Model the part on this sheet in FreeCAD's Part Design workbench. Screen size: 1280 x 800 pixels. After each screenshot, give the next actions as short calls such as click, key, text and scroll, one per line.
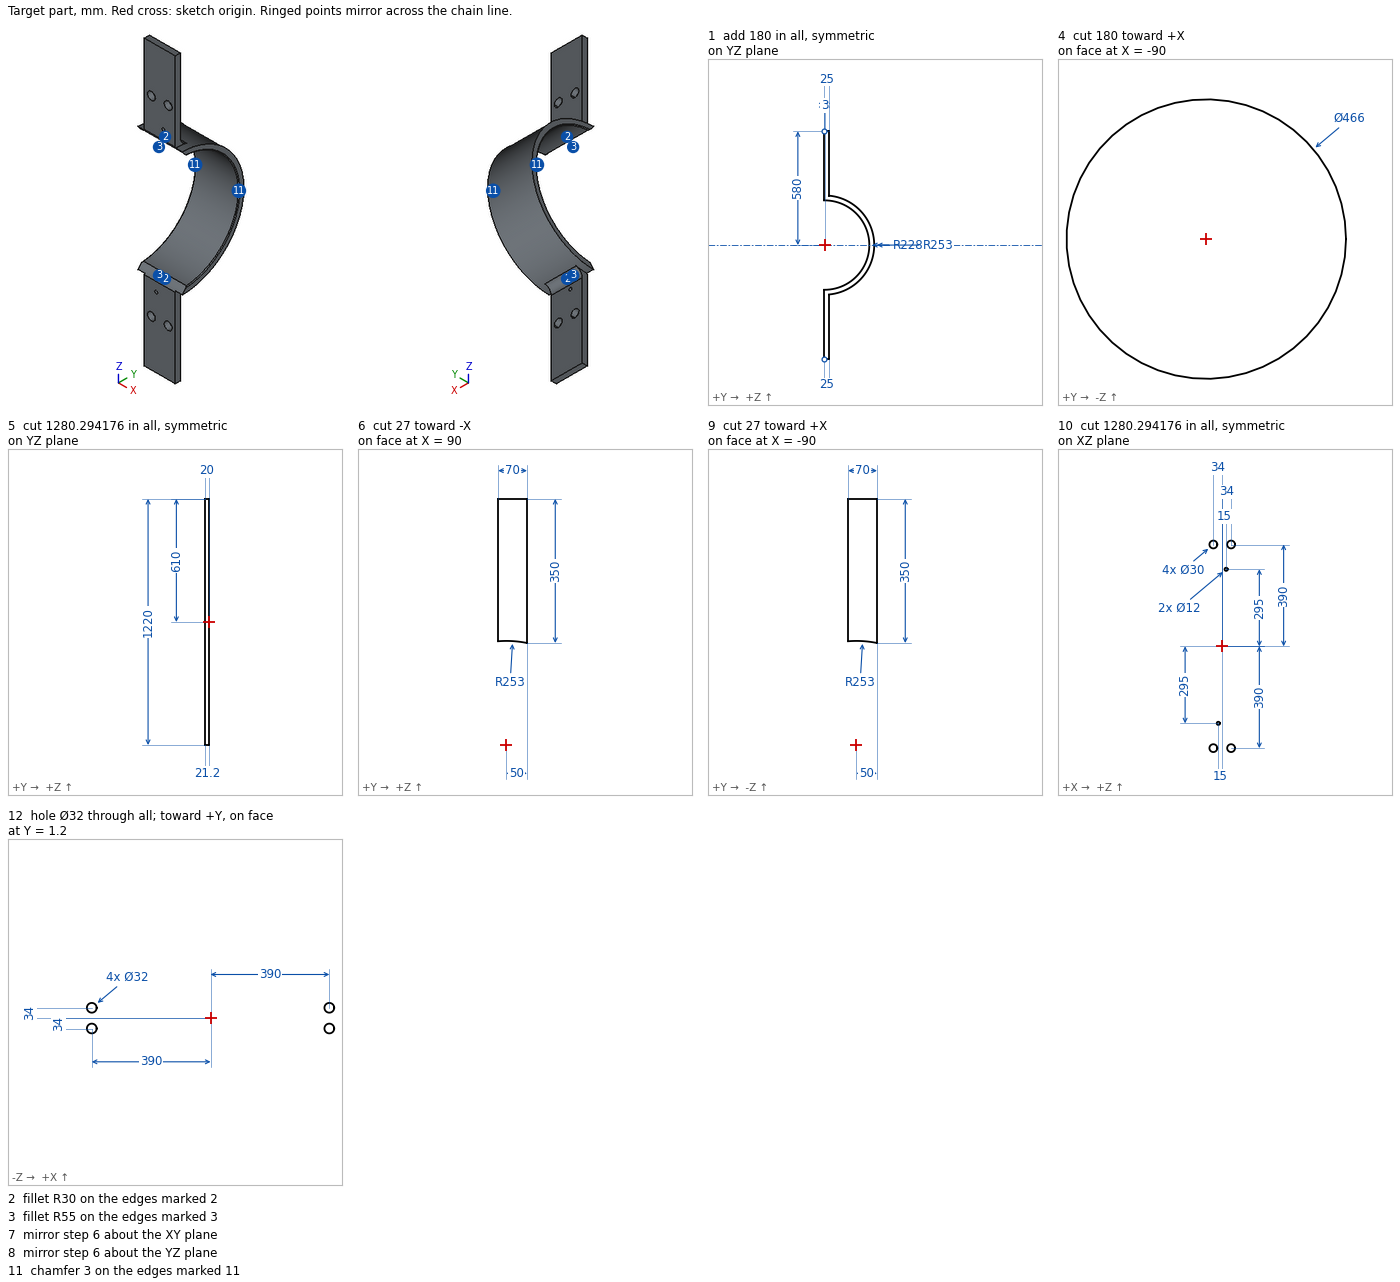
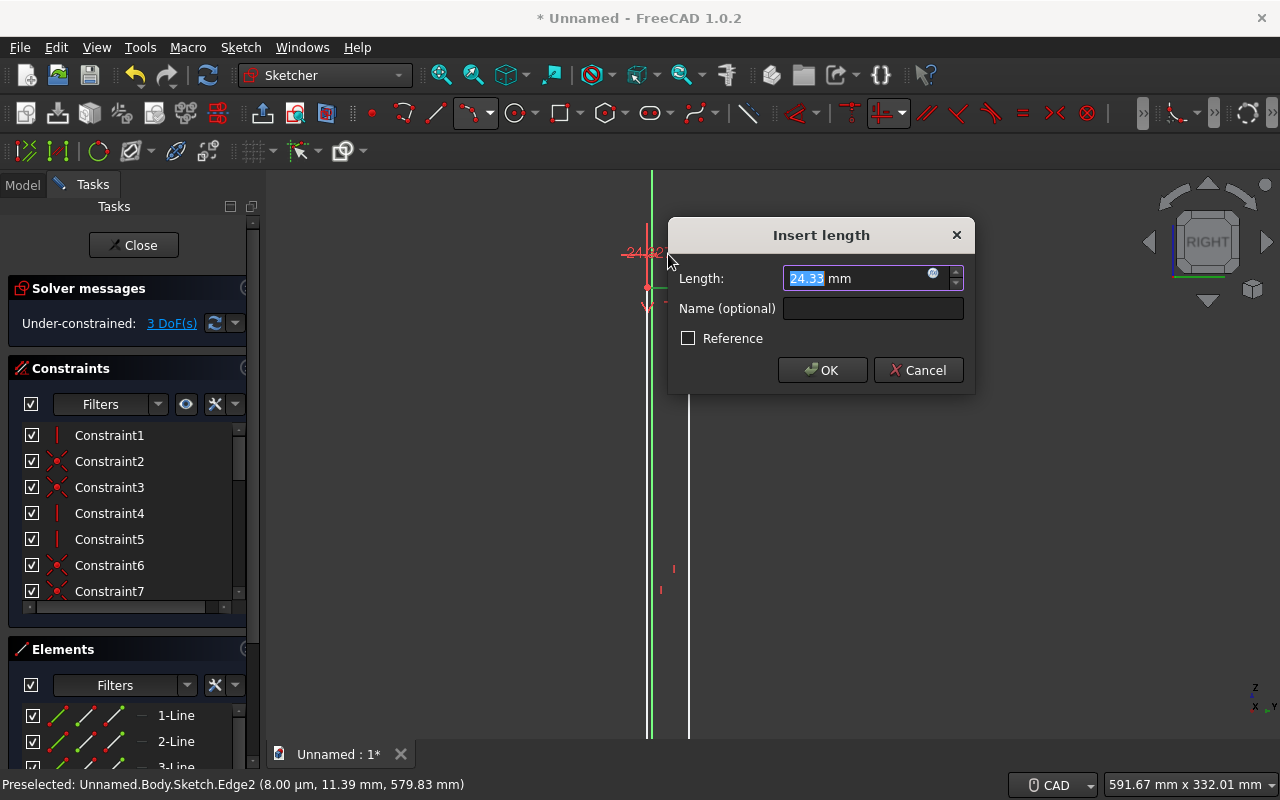
text(25)
key(Return)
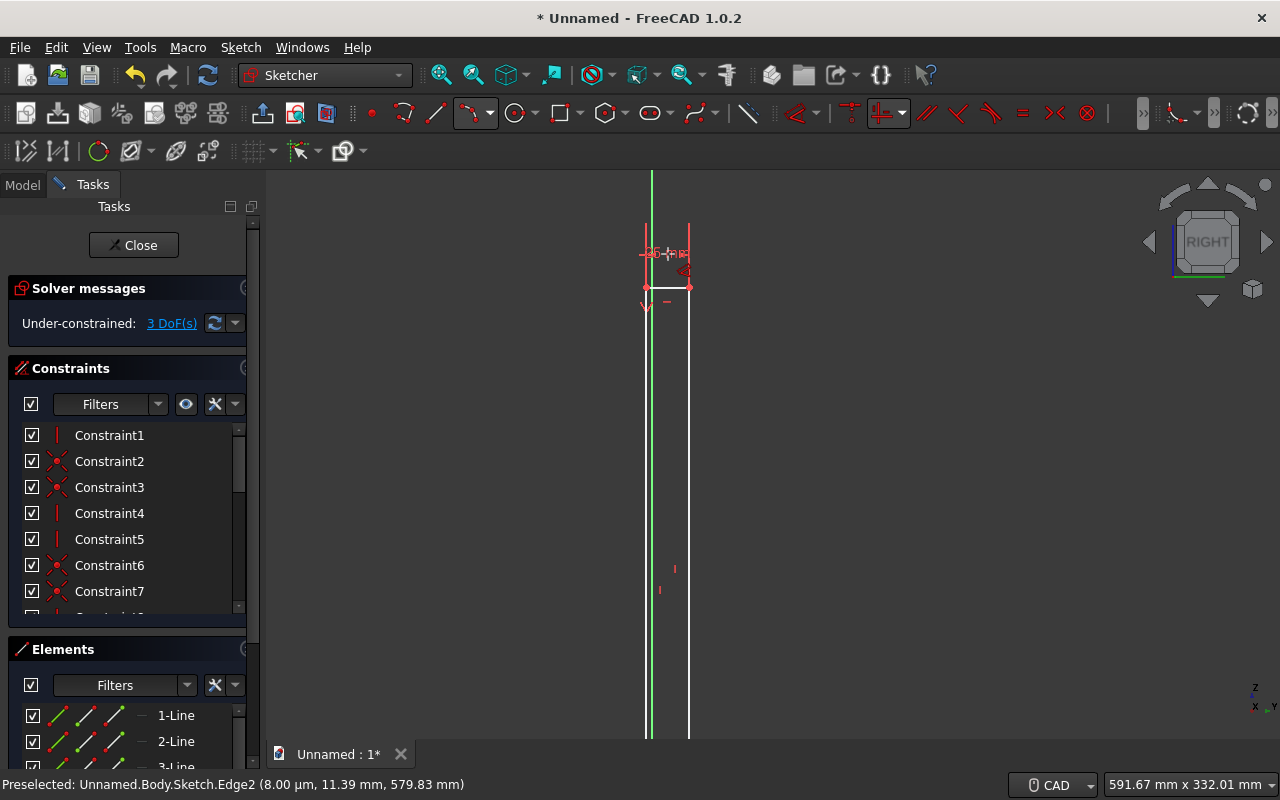
scroll(672, 291, down, 9)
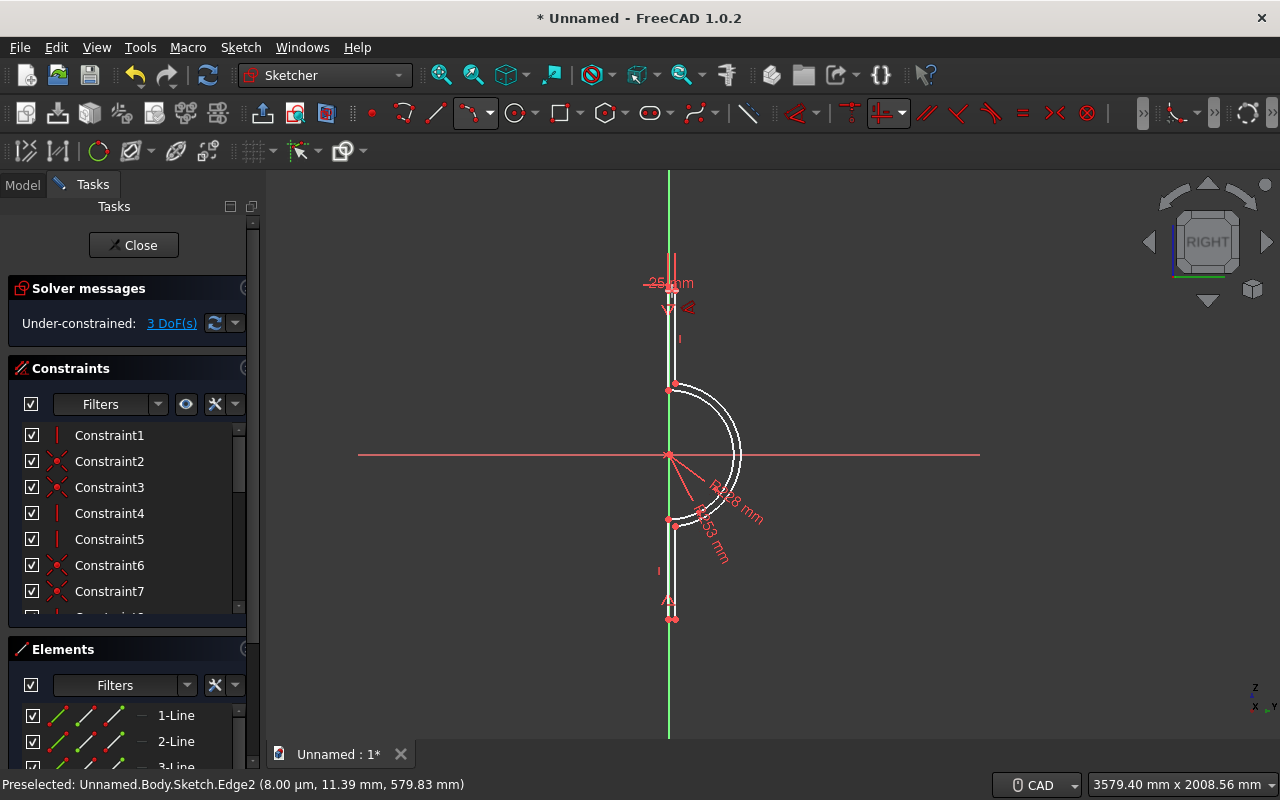
scroll(673, 619, up, 10)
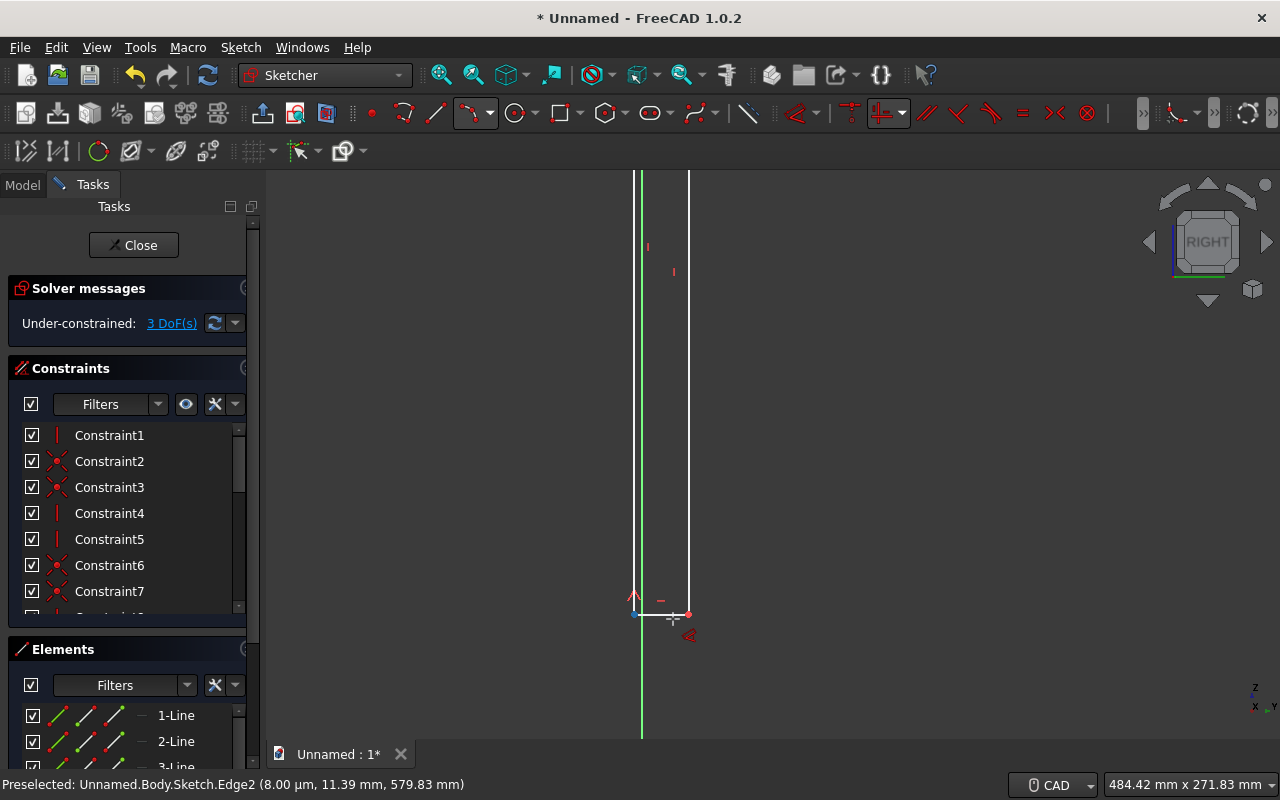
click(672, 615)
click(661, 649)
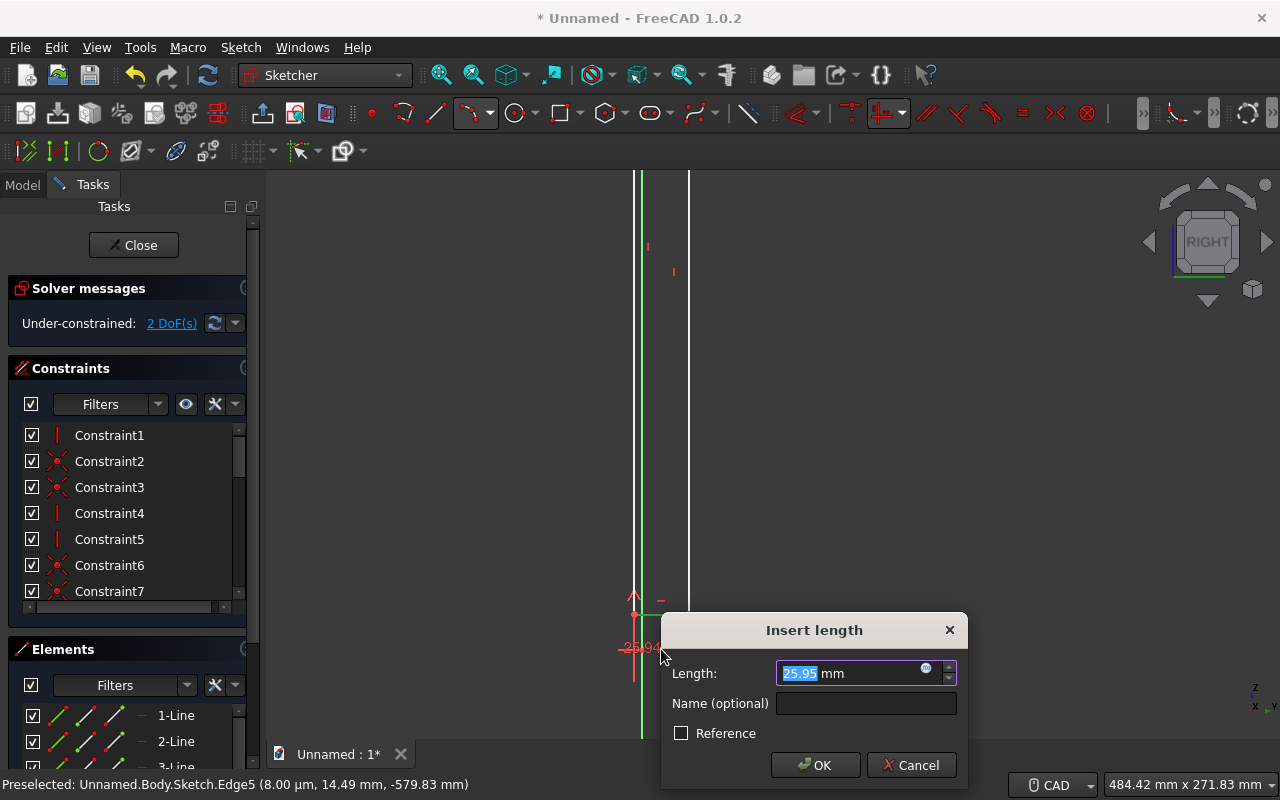
text(25)
key(Return)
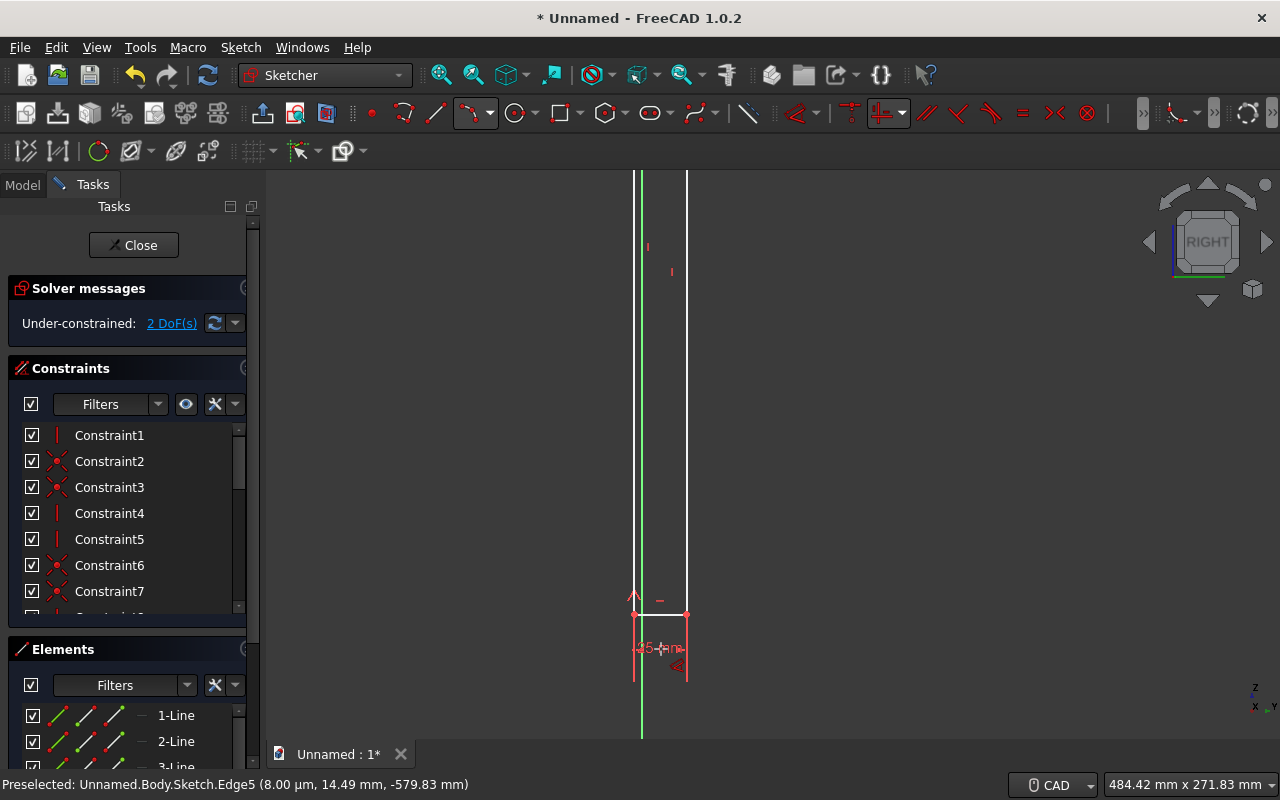
scroll(673, 619, down, 10)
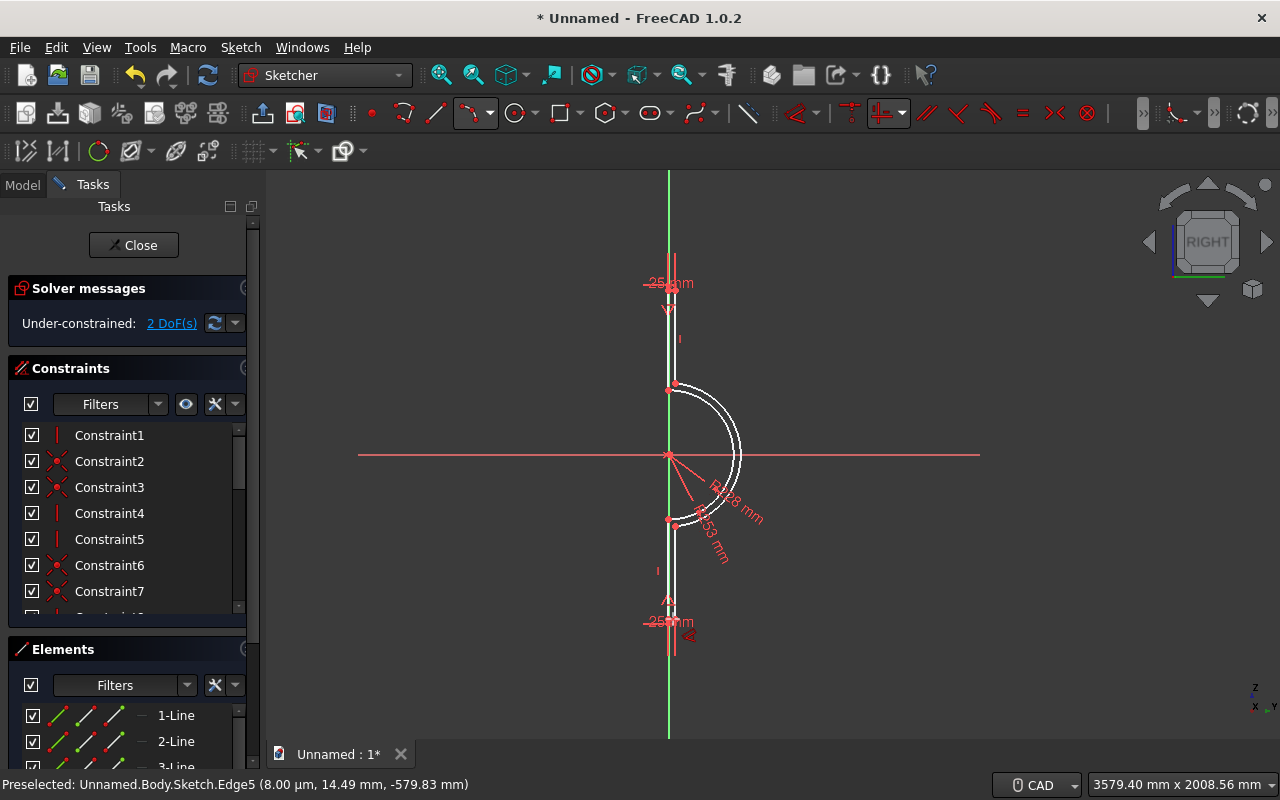
scroll(668, 291, up, 20)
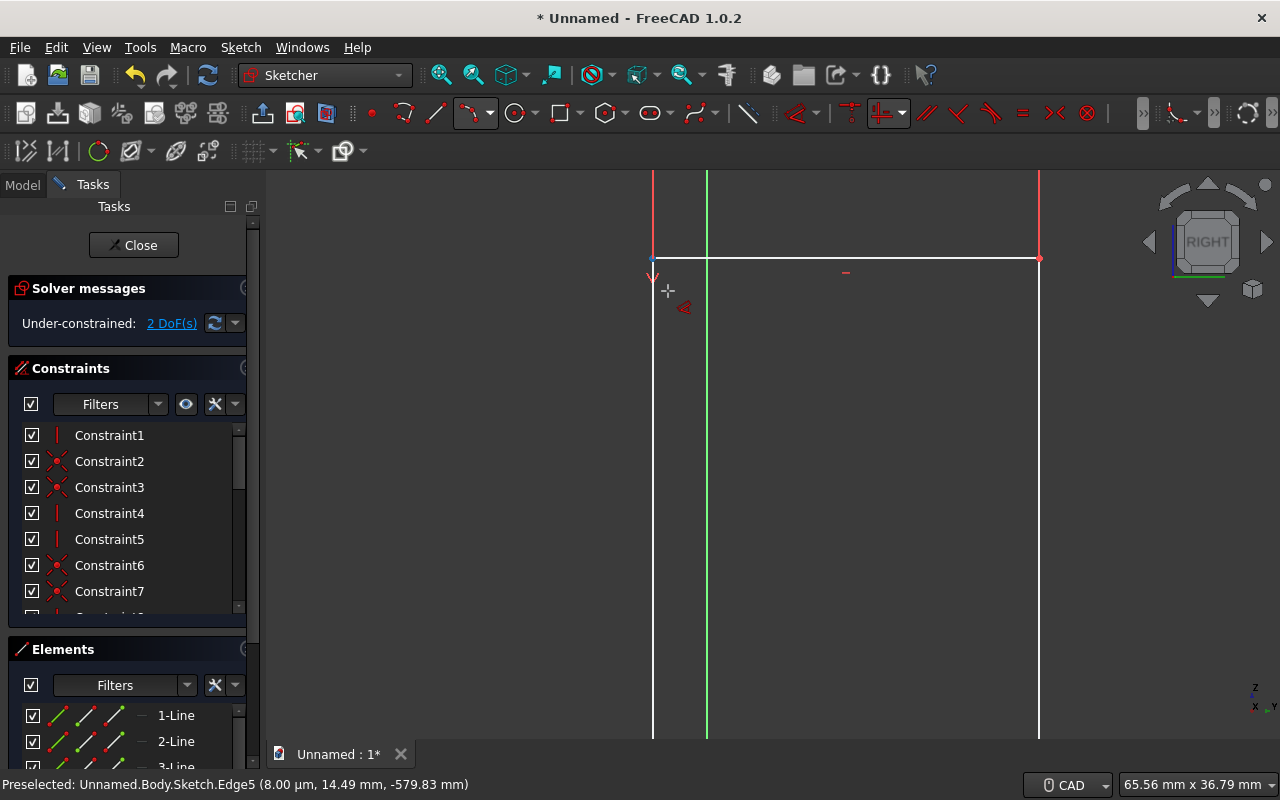
click(653, 258)
click(680, 224)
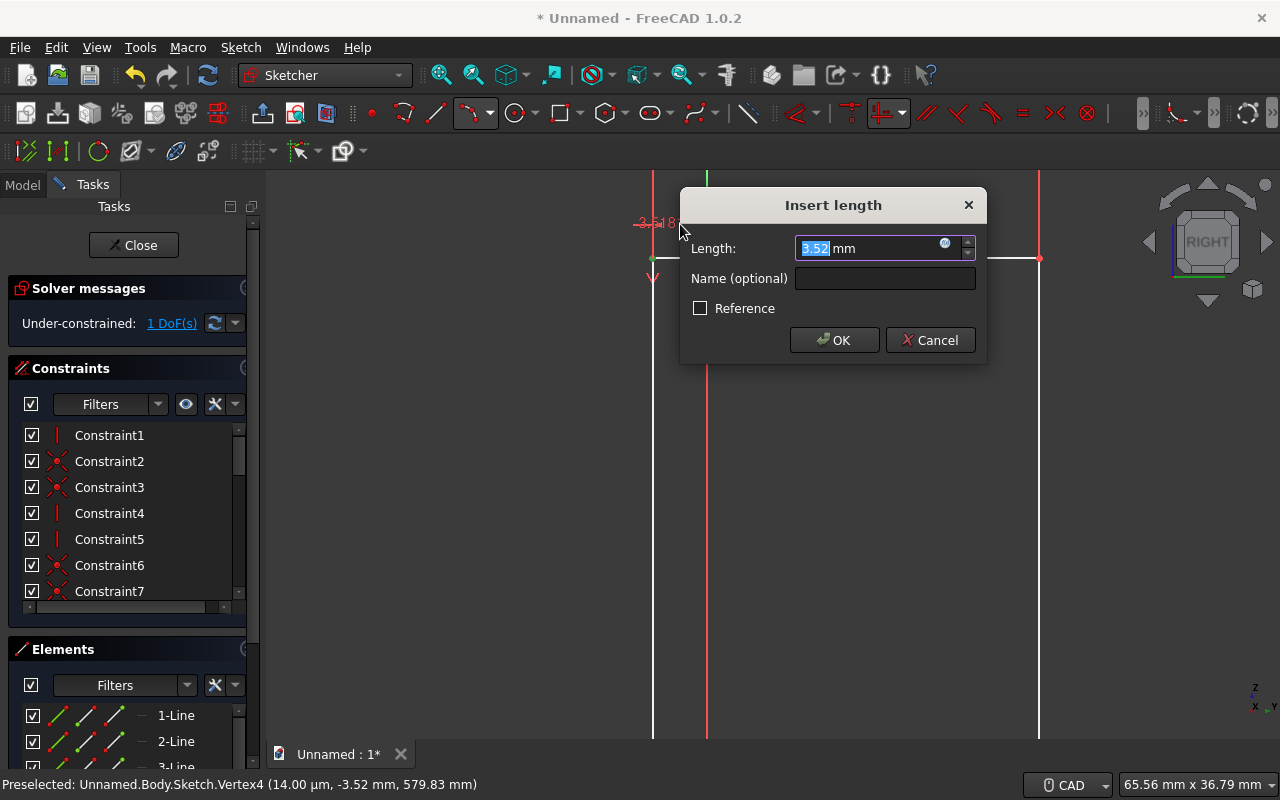
text(3)
key(Return)